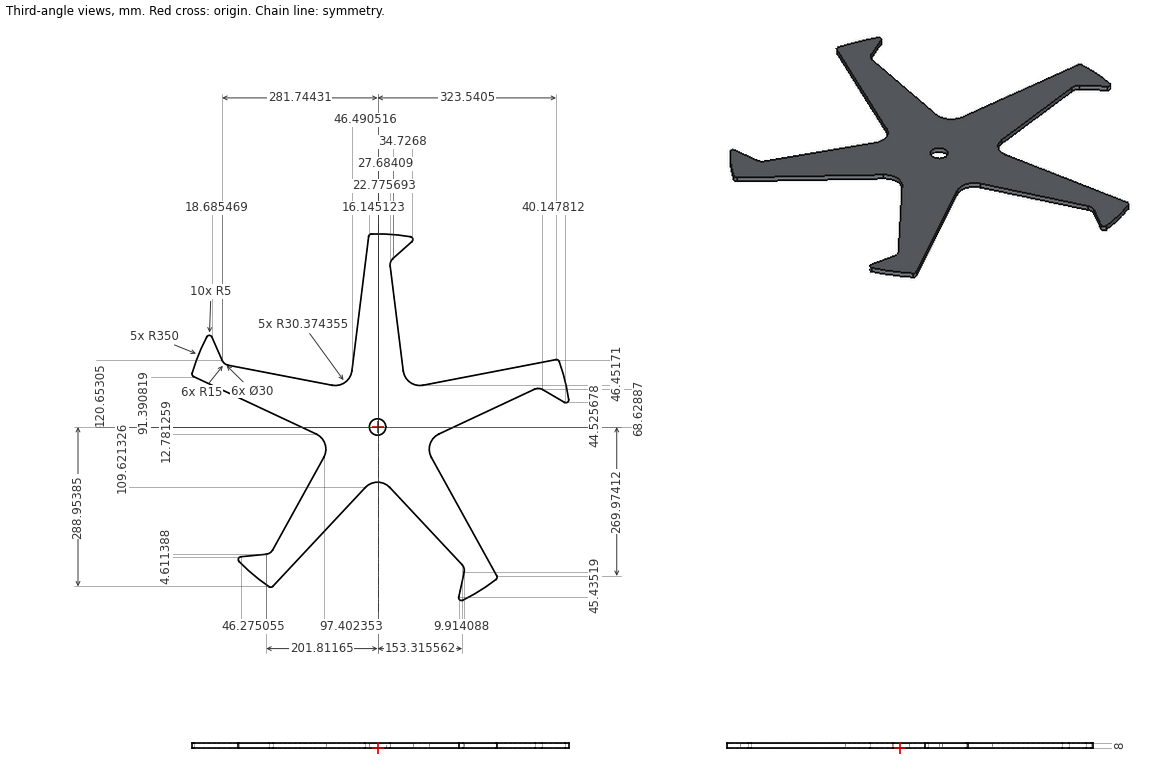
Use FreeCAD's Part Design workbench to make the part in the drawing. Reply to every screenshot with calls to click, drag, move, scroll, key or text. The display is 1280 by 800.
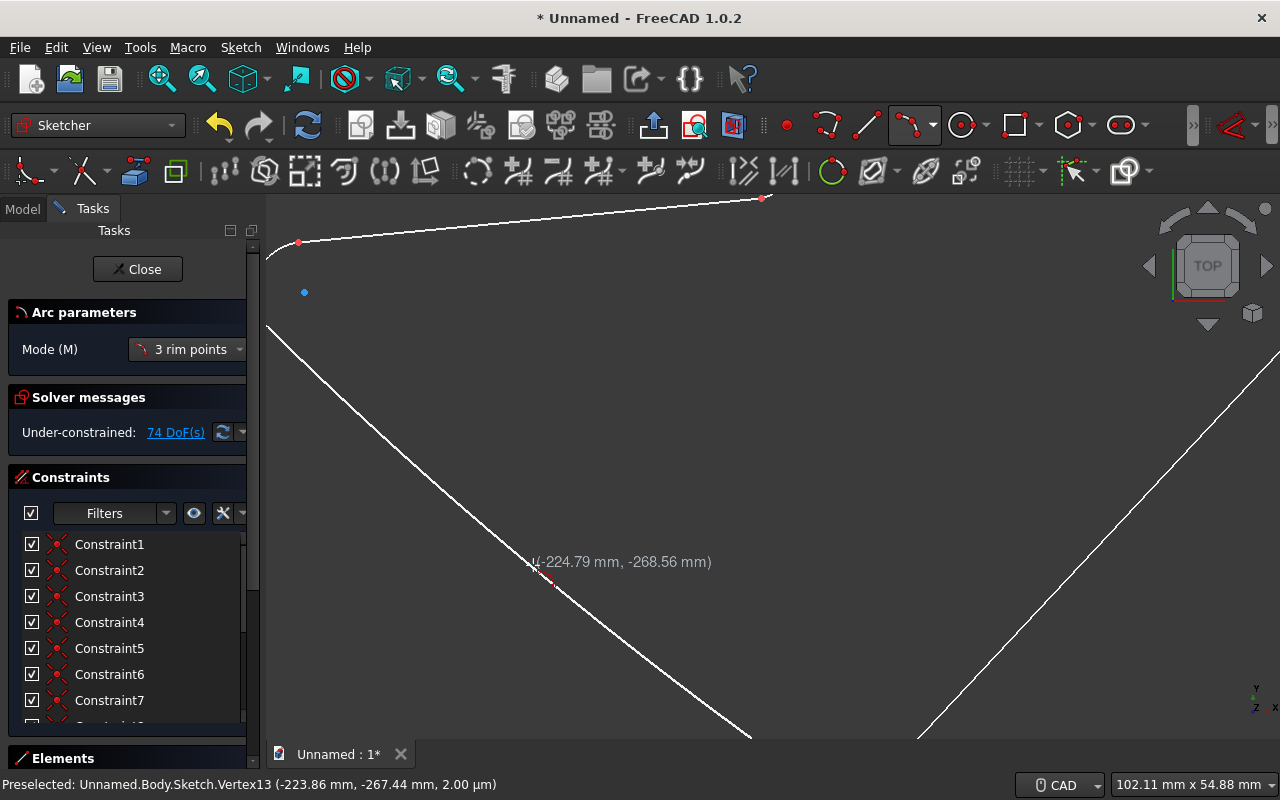
click(530, 563)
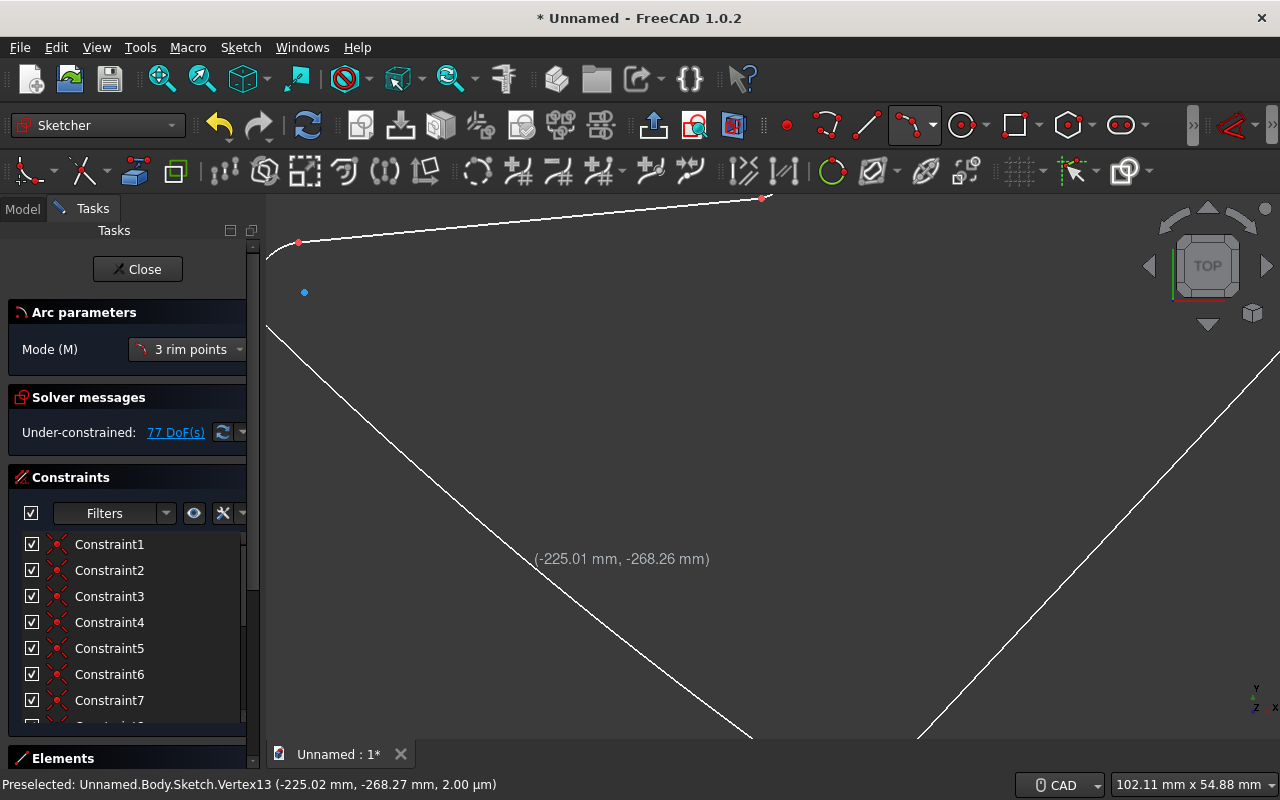
scroll(594, 610, down, 15)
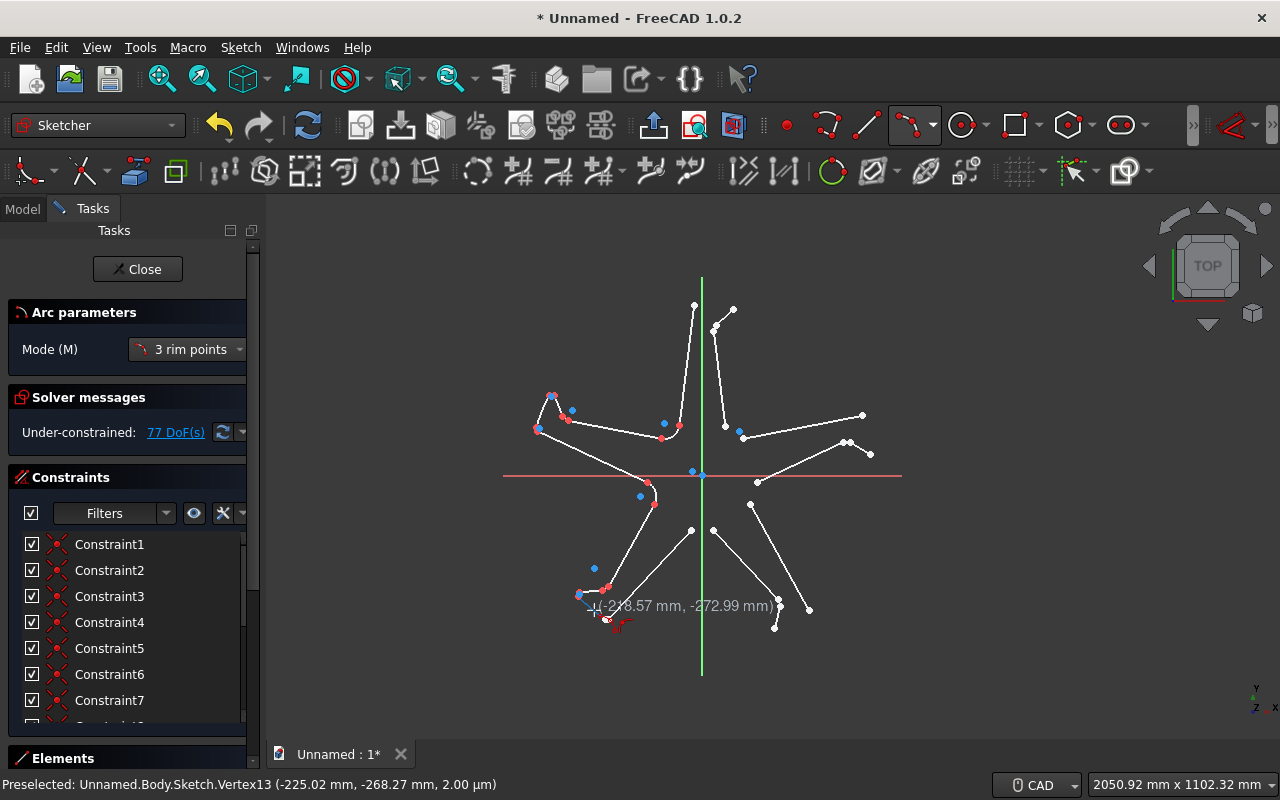
scroll(605, 619, up, 8)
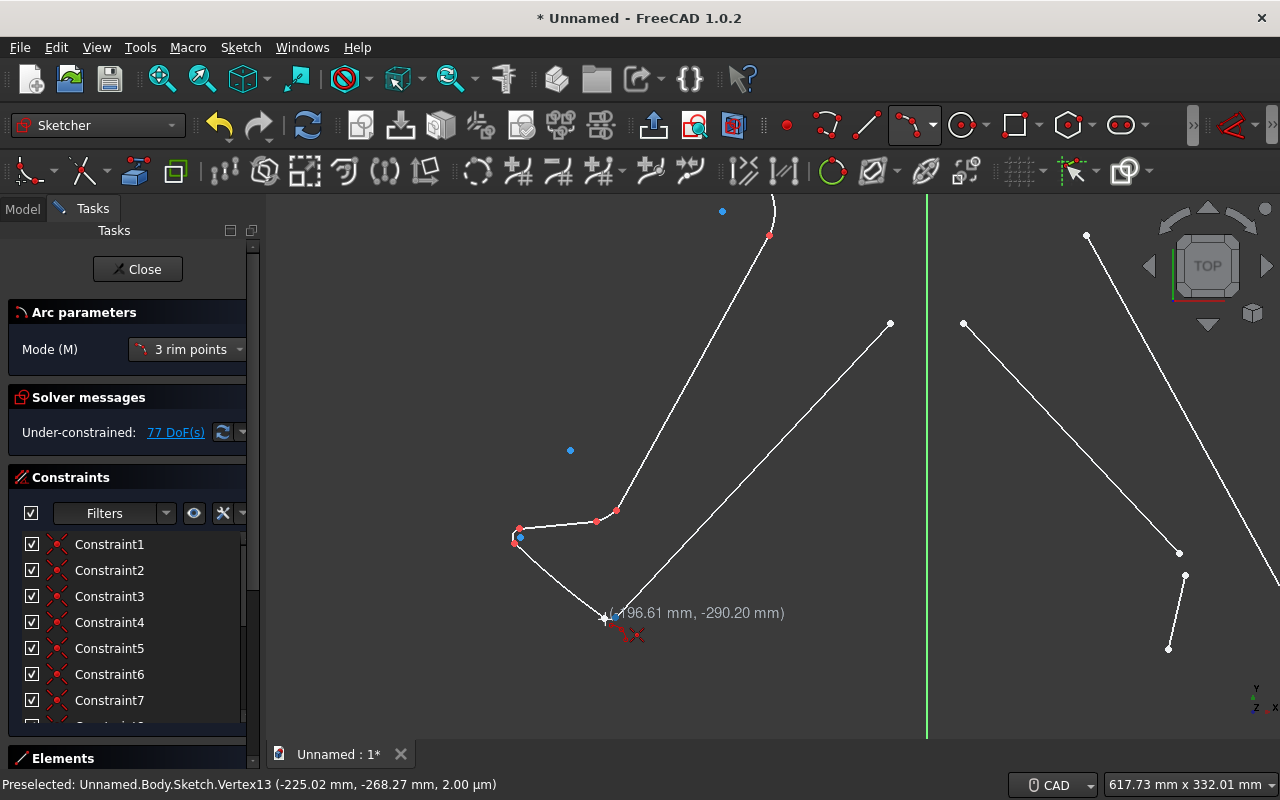
click(604, 617)
click(621, 617)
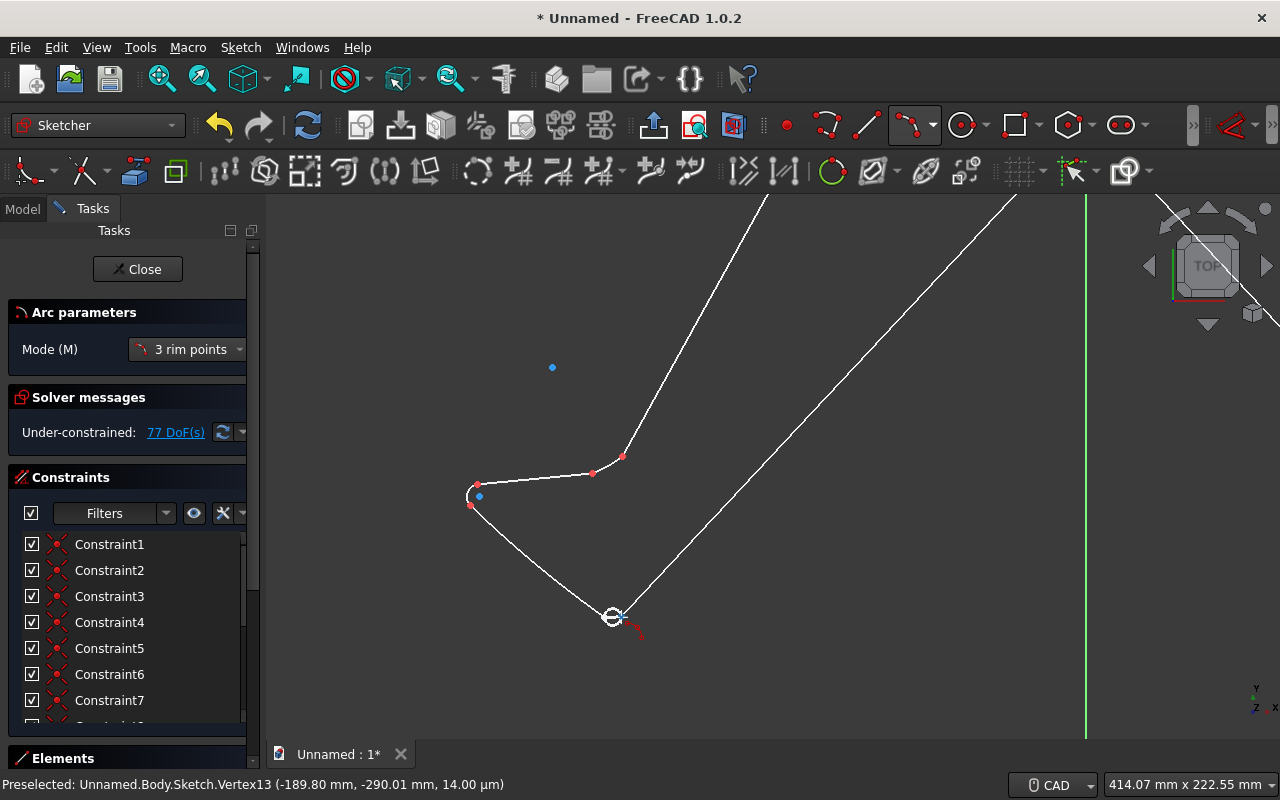
scroll(613, 618, up, 9)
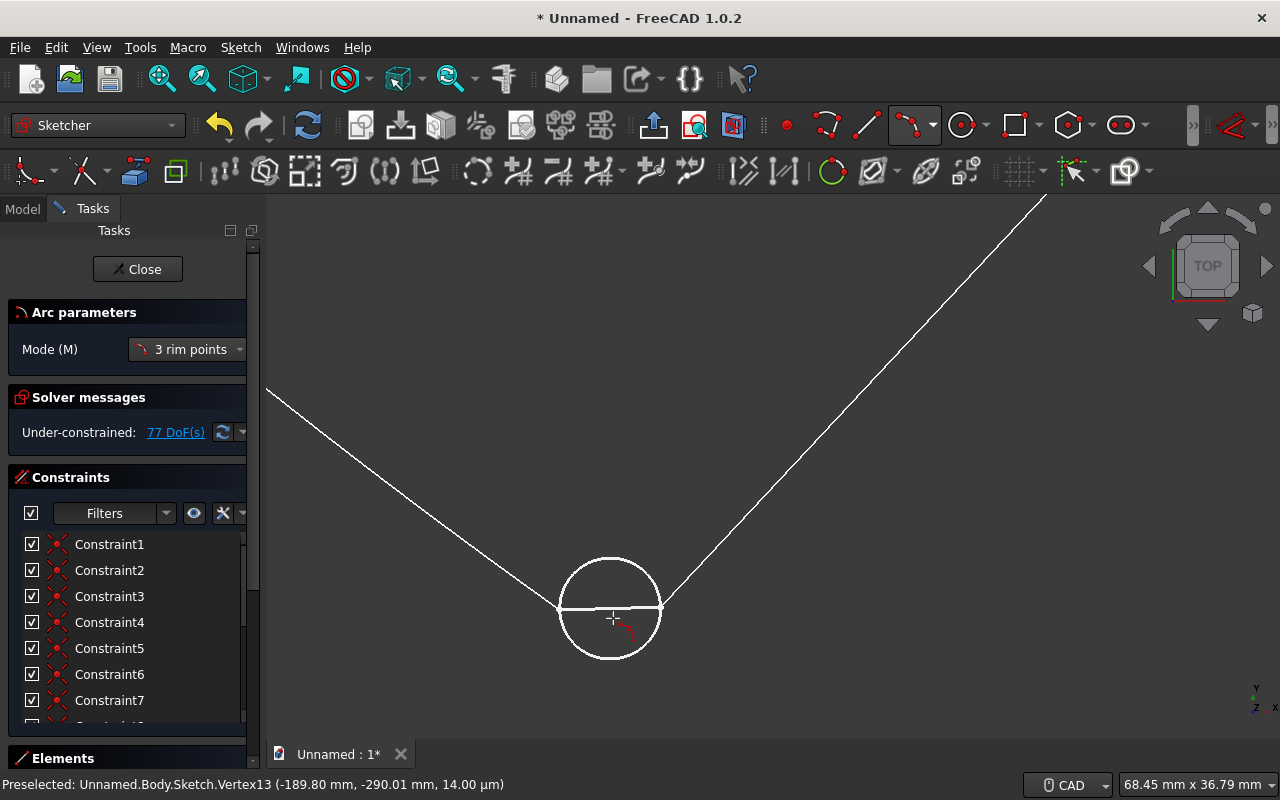
click(612, 614)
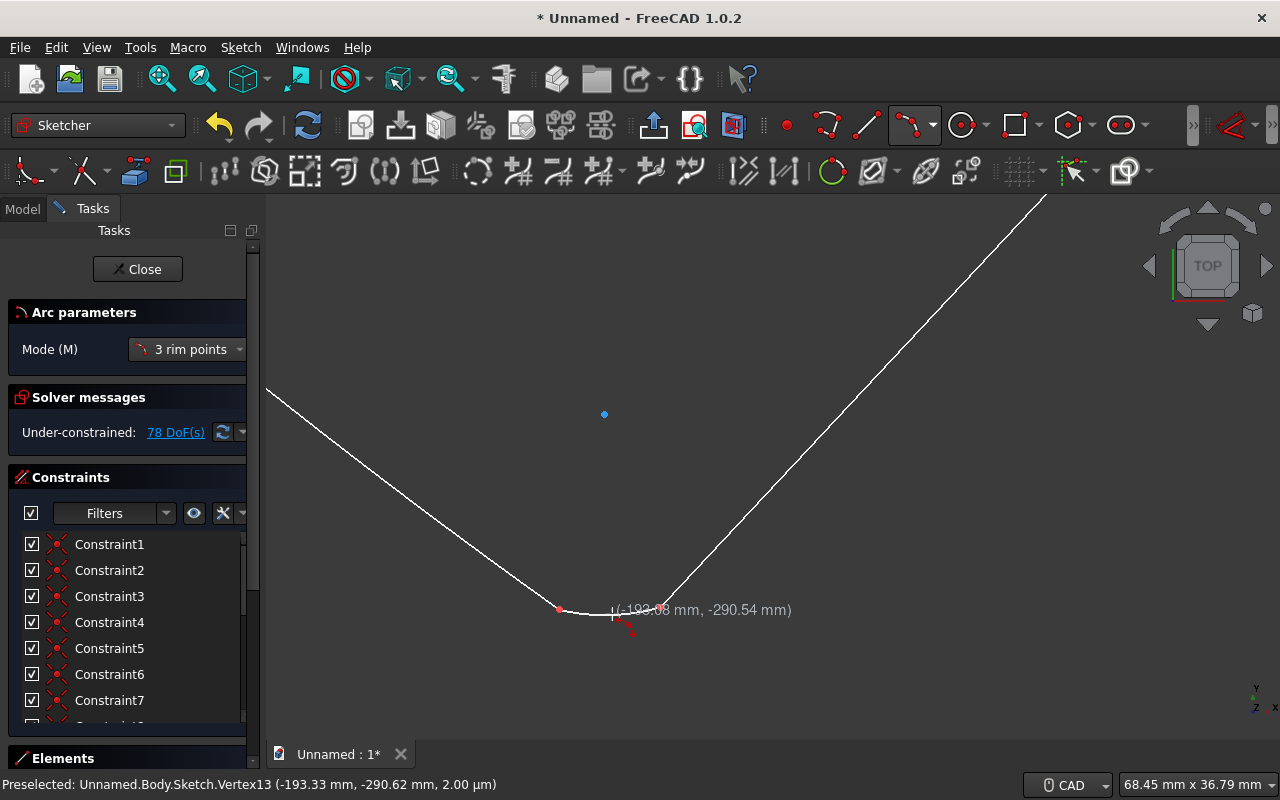
scroll(584, 654, down, 16)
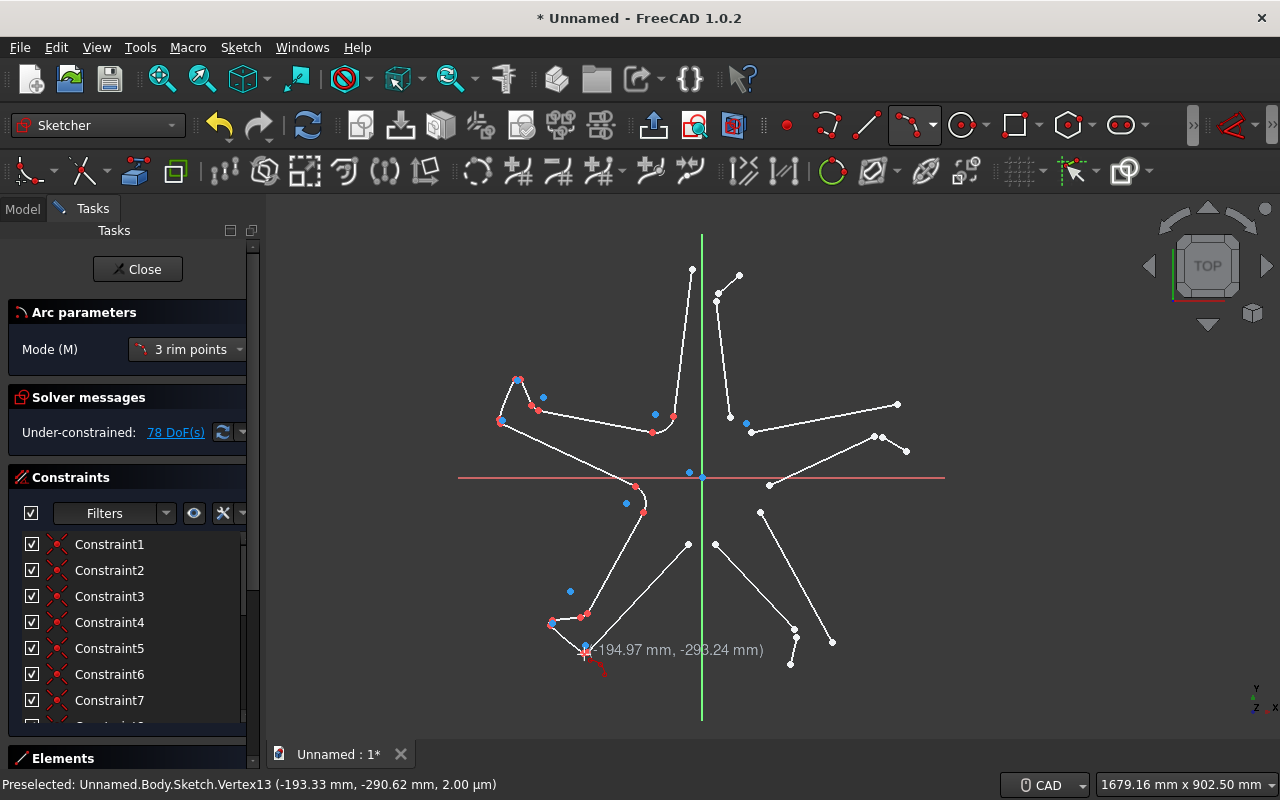
click(689, 545)
click(715, 545)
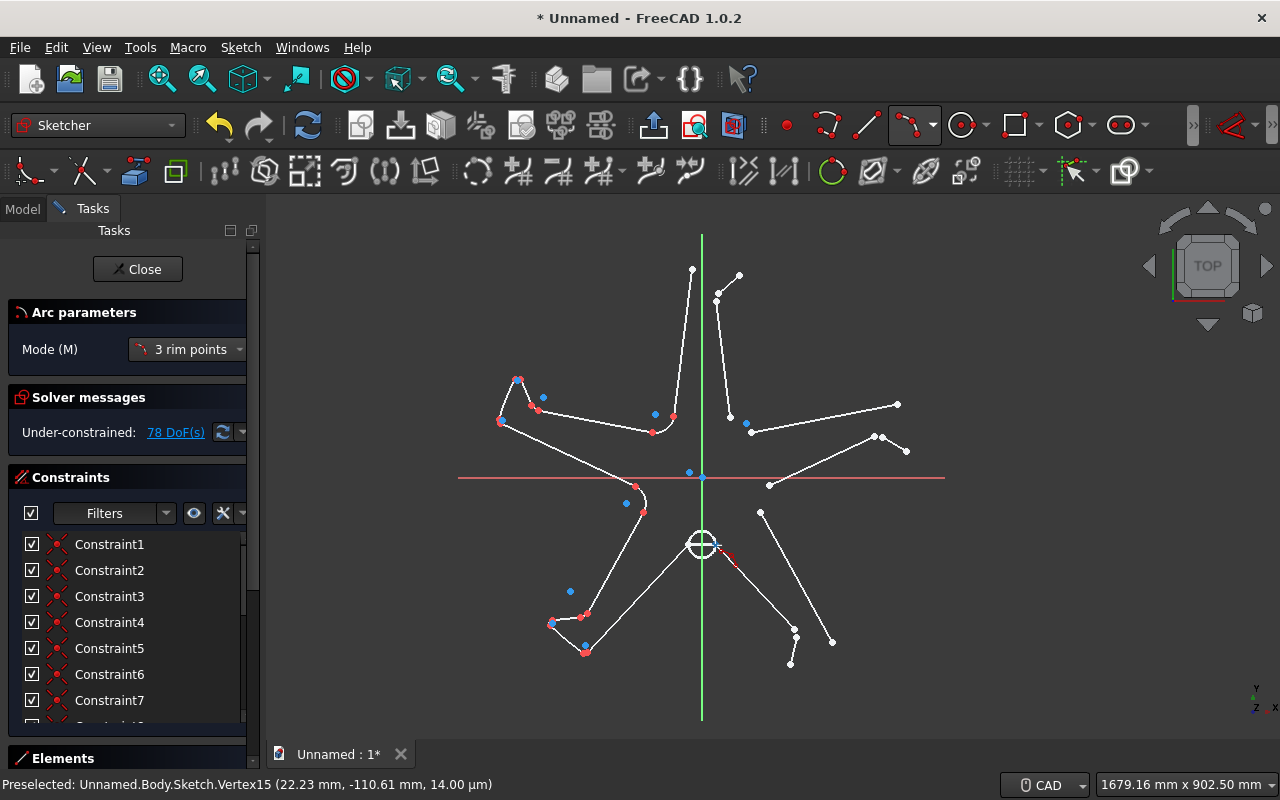
scroll(708, 539, up, 6)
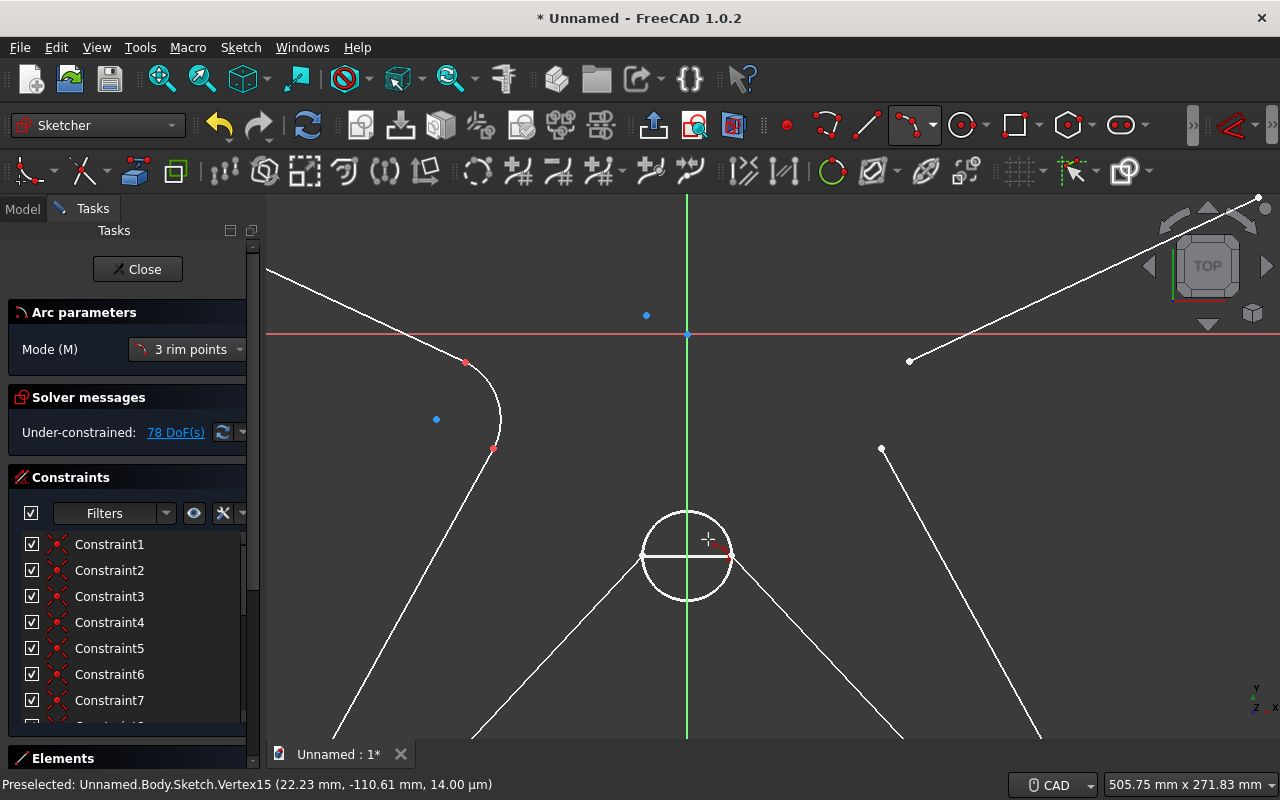
click(707, 538)